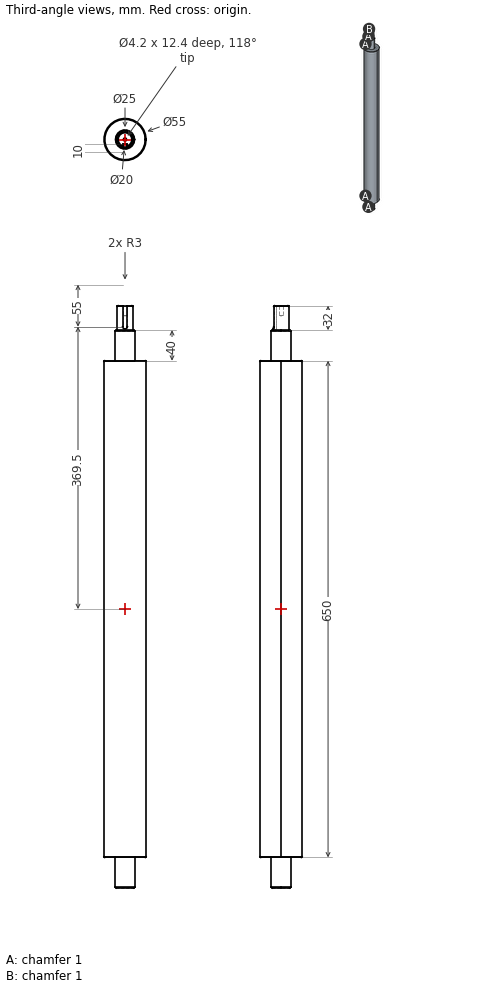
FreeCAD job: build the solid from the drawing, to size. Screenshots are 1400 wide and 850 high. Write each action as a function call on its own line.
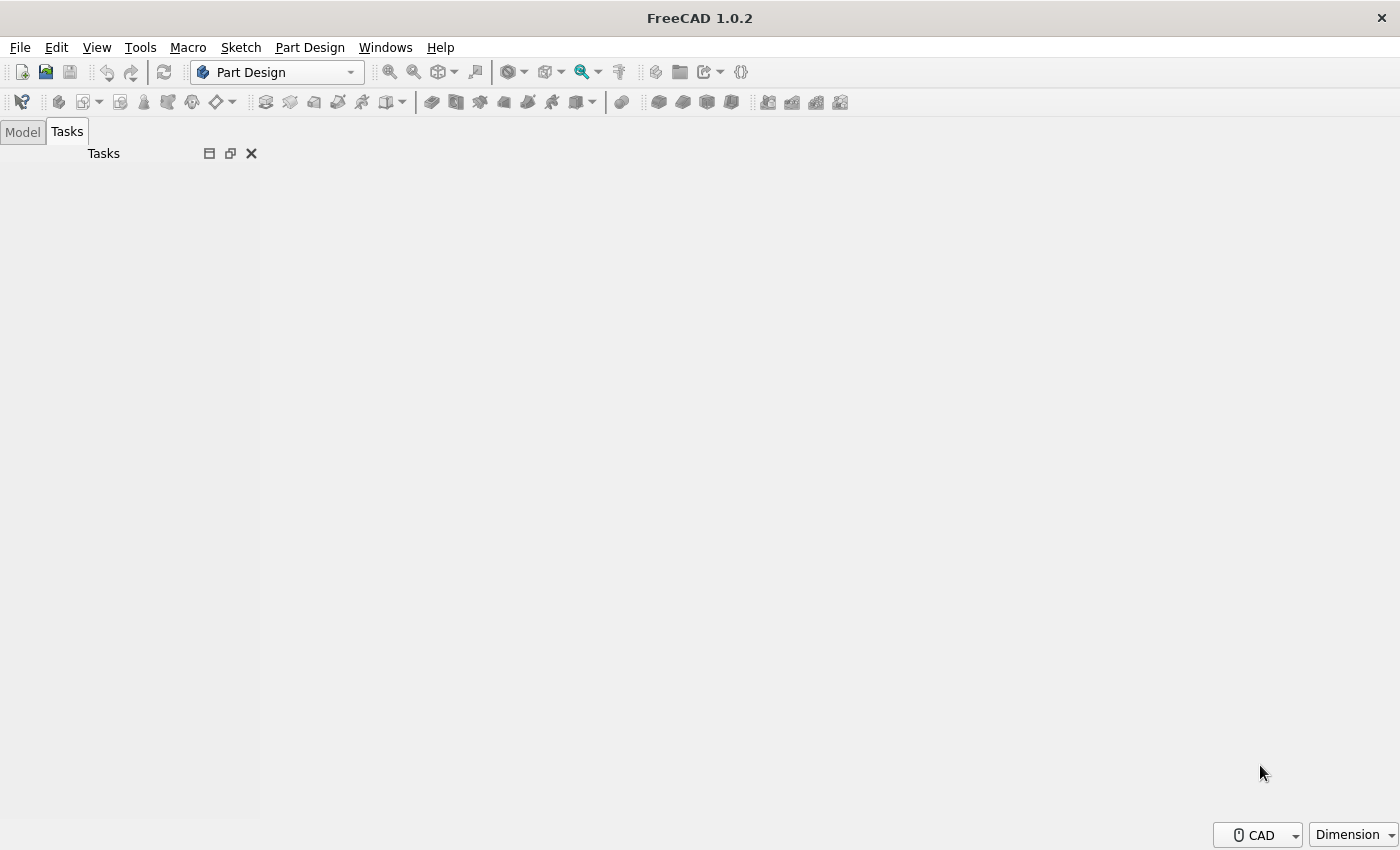
click(22, 72)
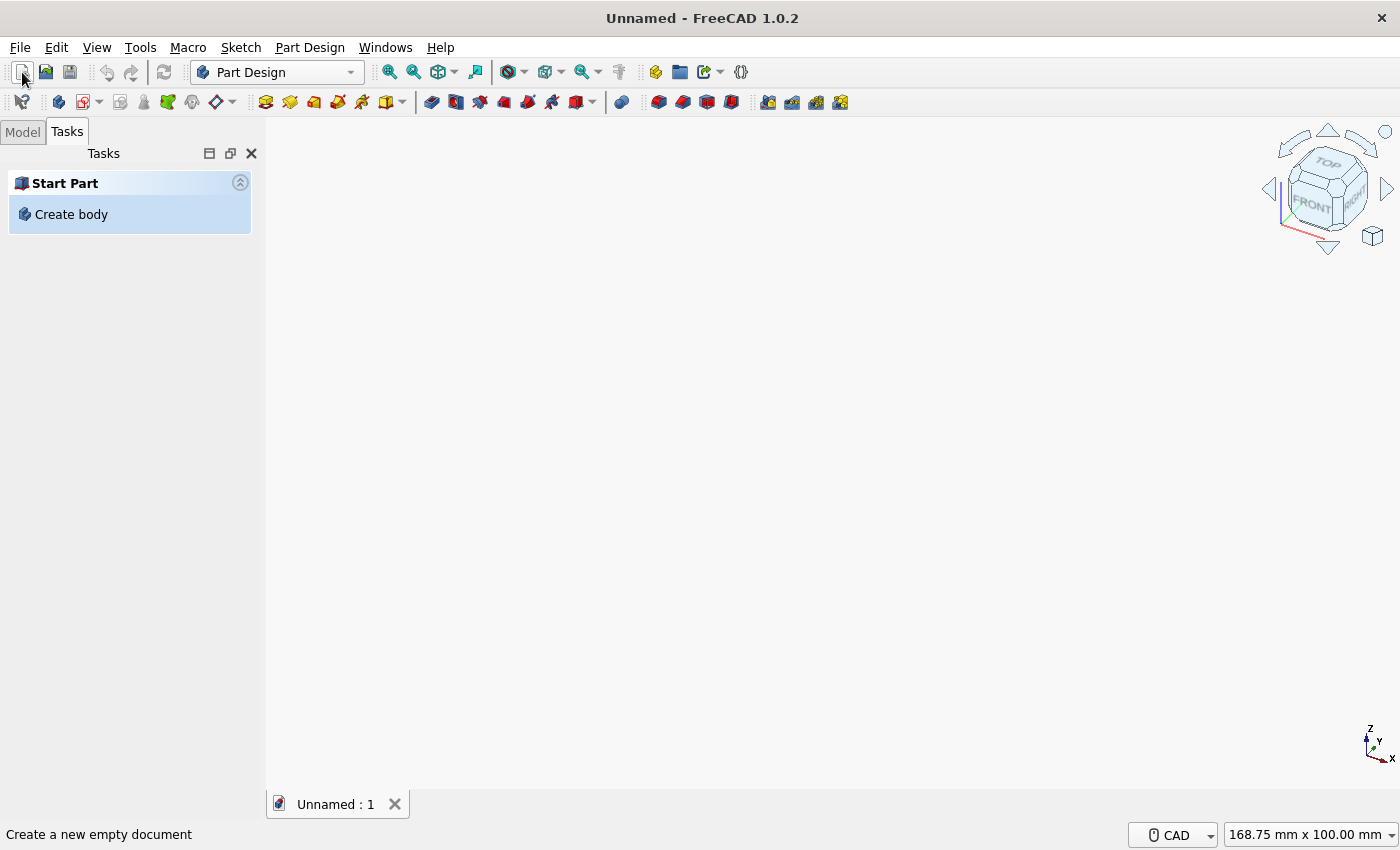
click(84, 102)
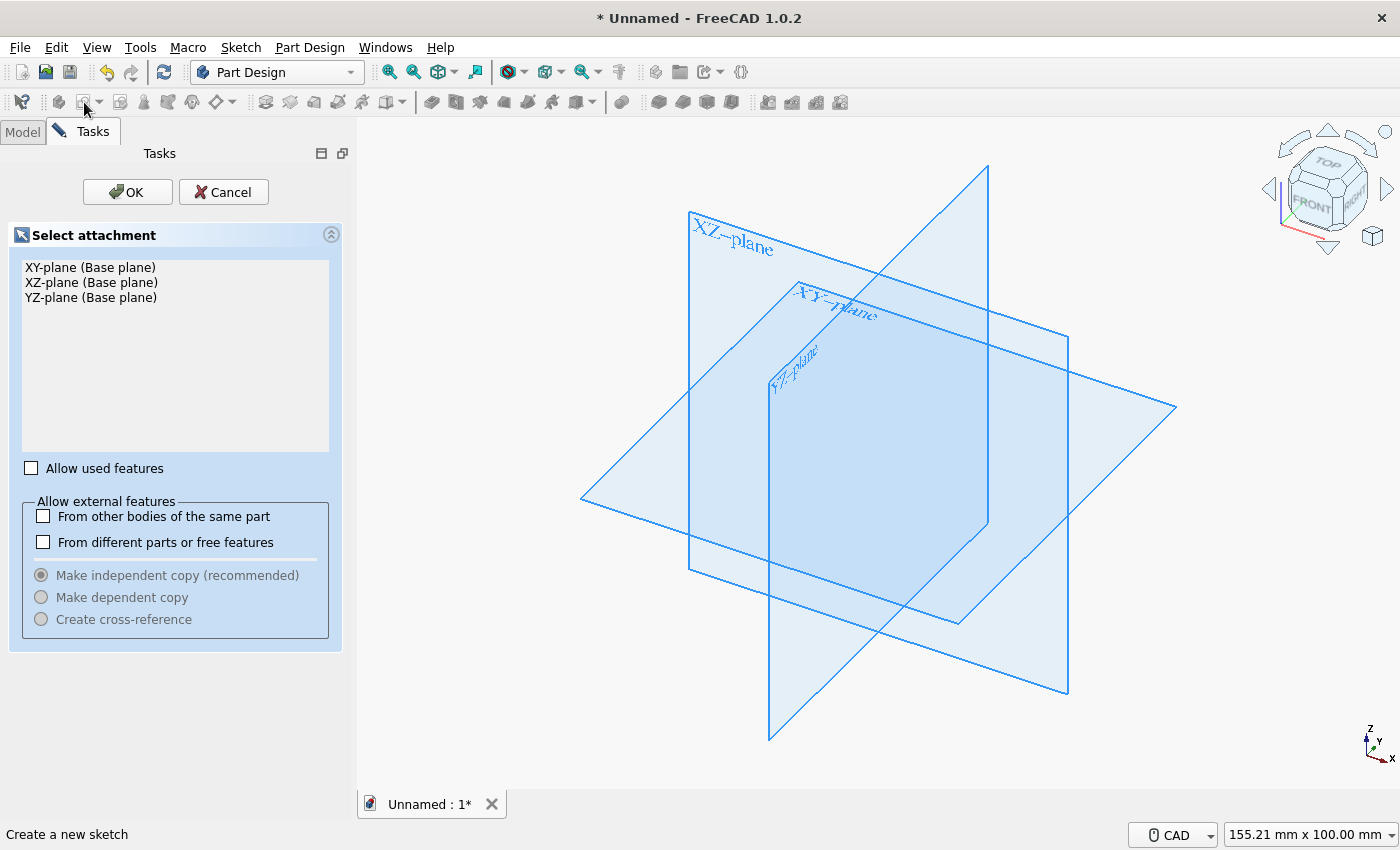
click(82, 268)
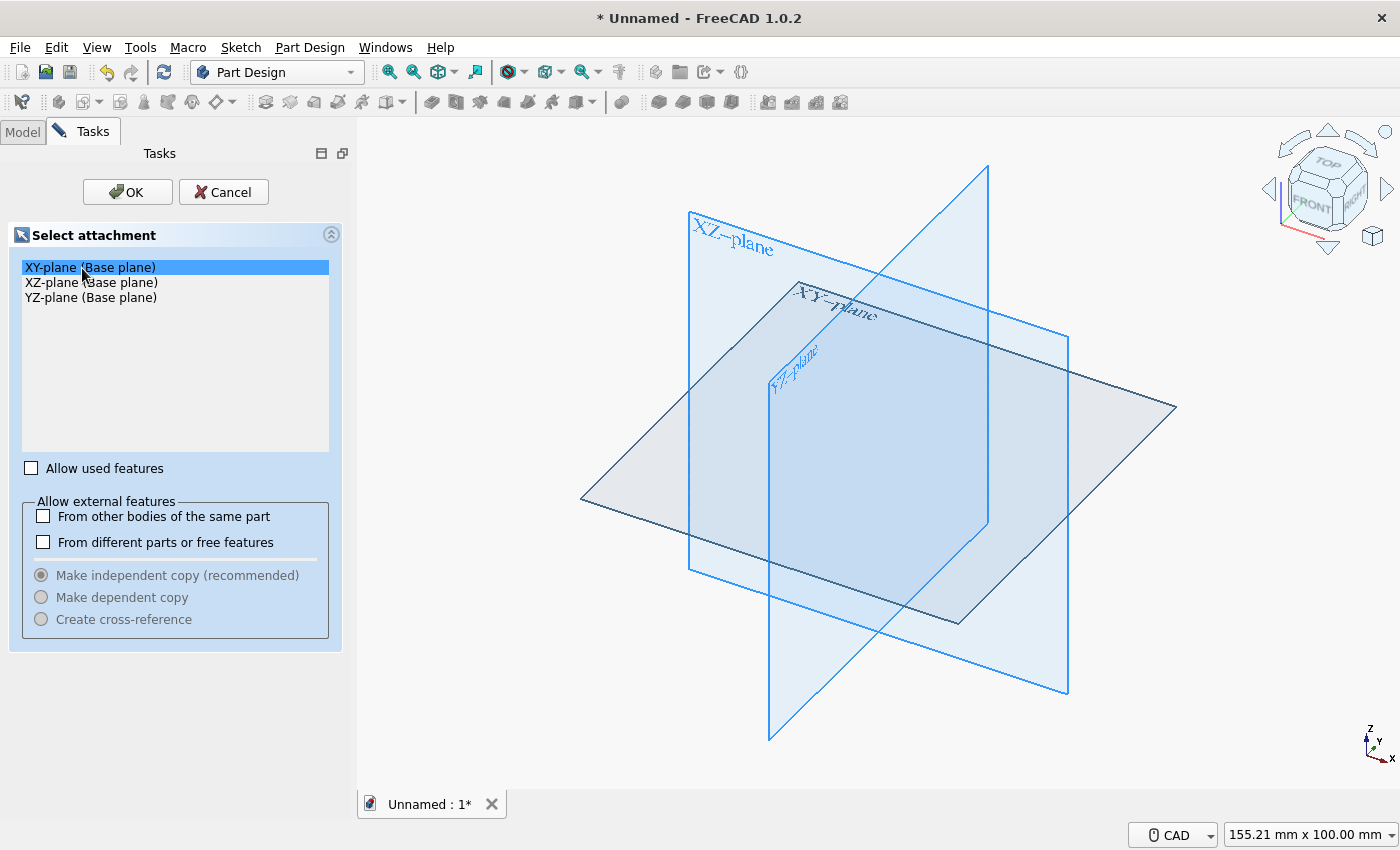
click(128, 192)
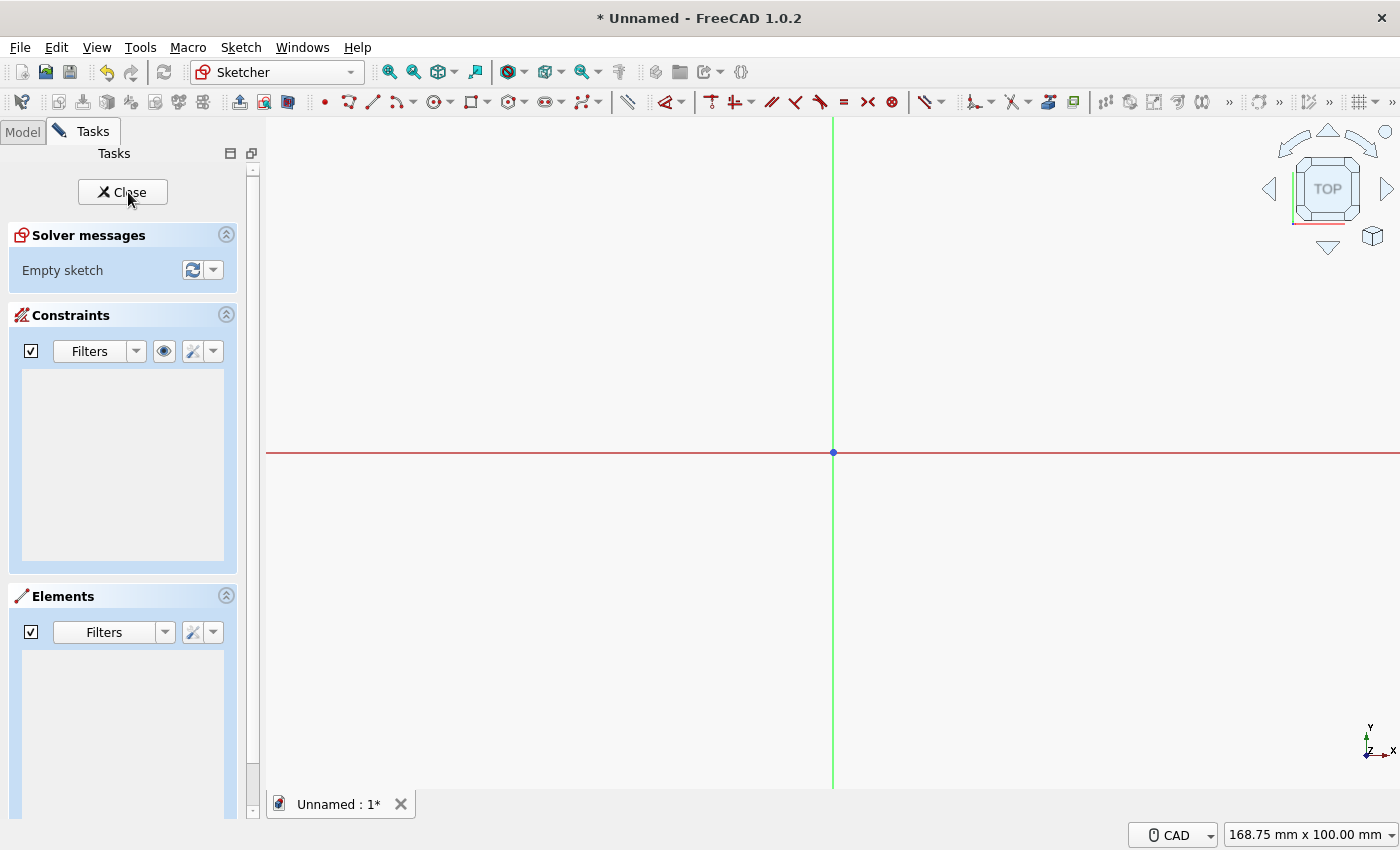
click(434, 102)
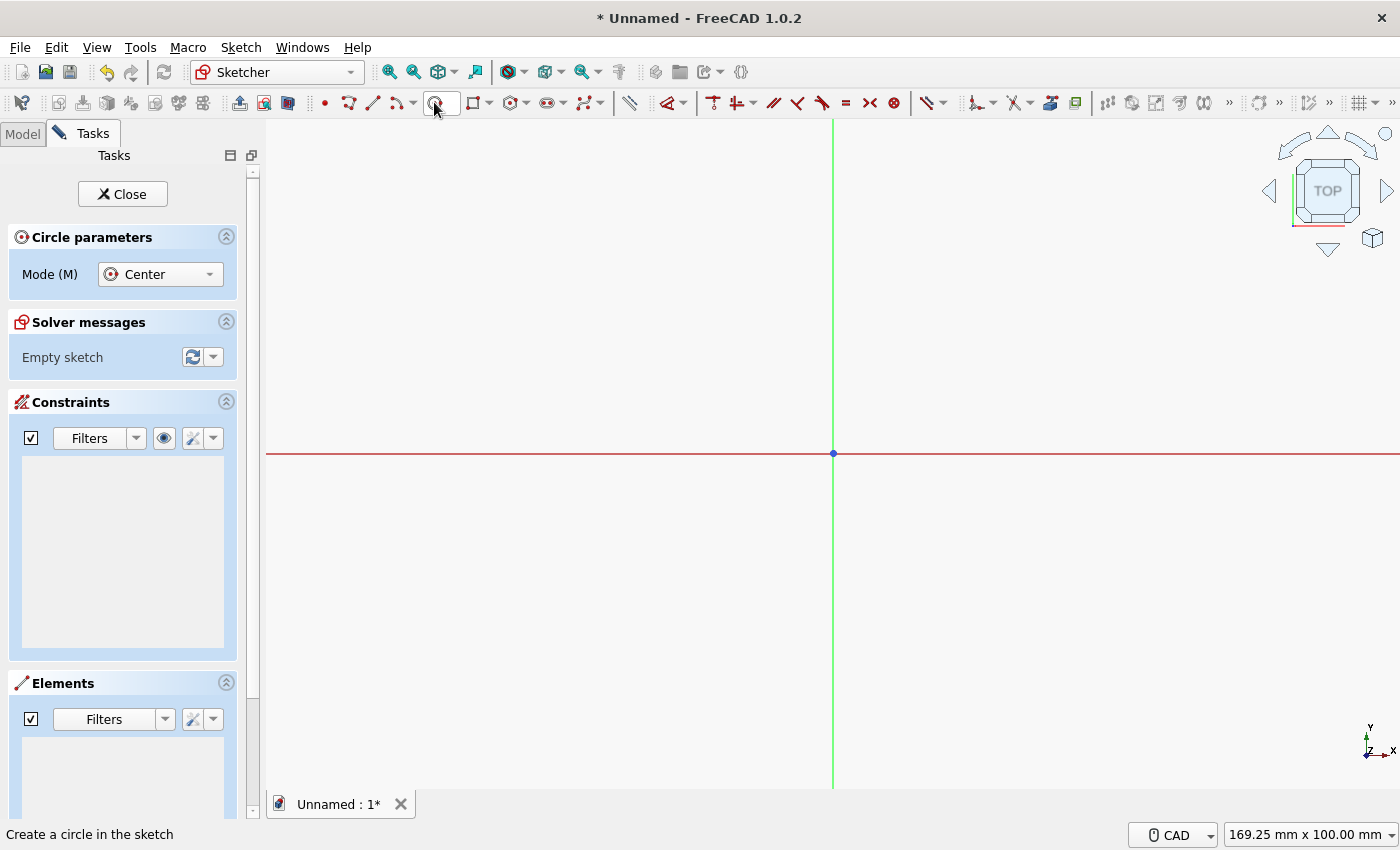
click(833, 454)
move(963, 324)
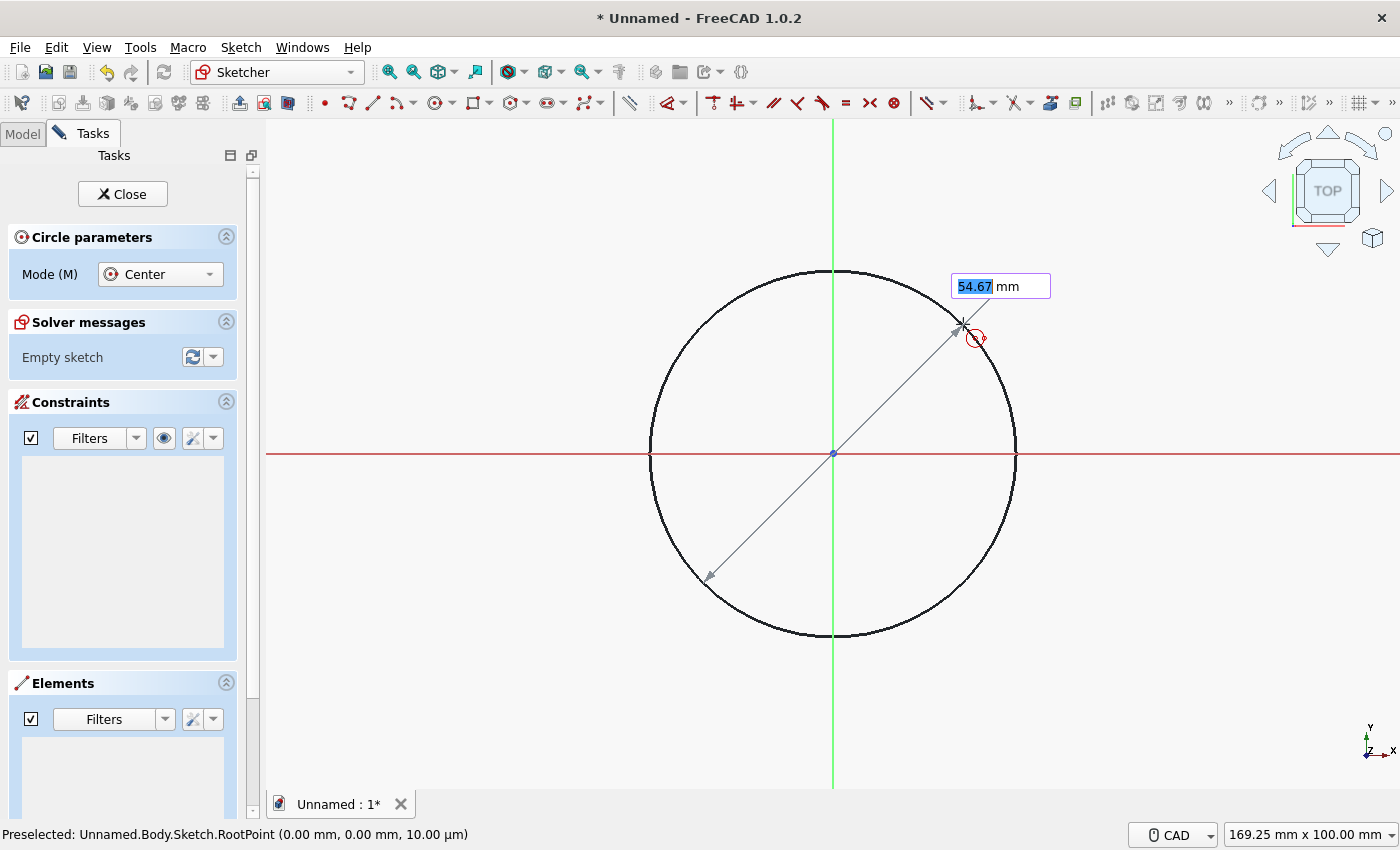
text(55)
key(Return)
key(Escape)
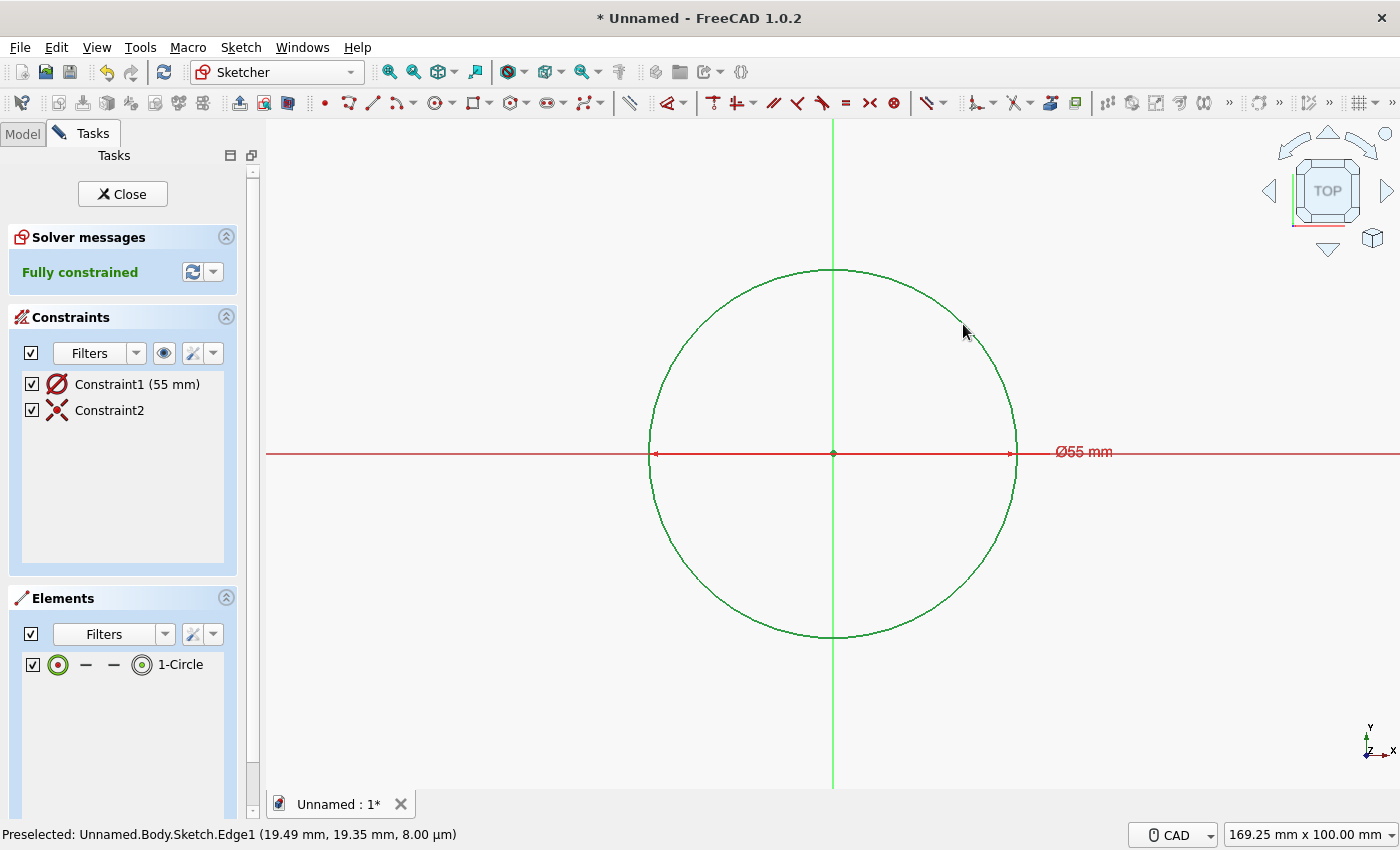
click(123, 194)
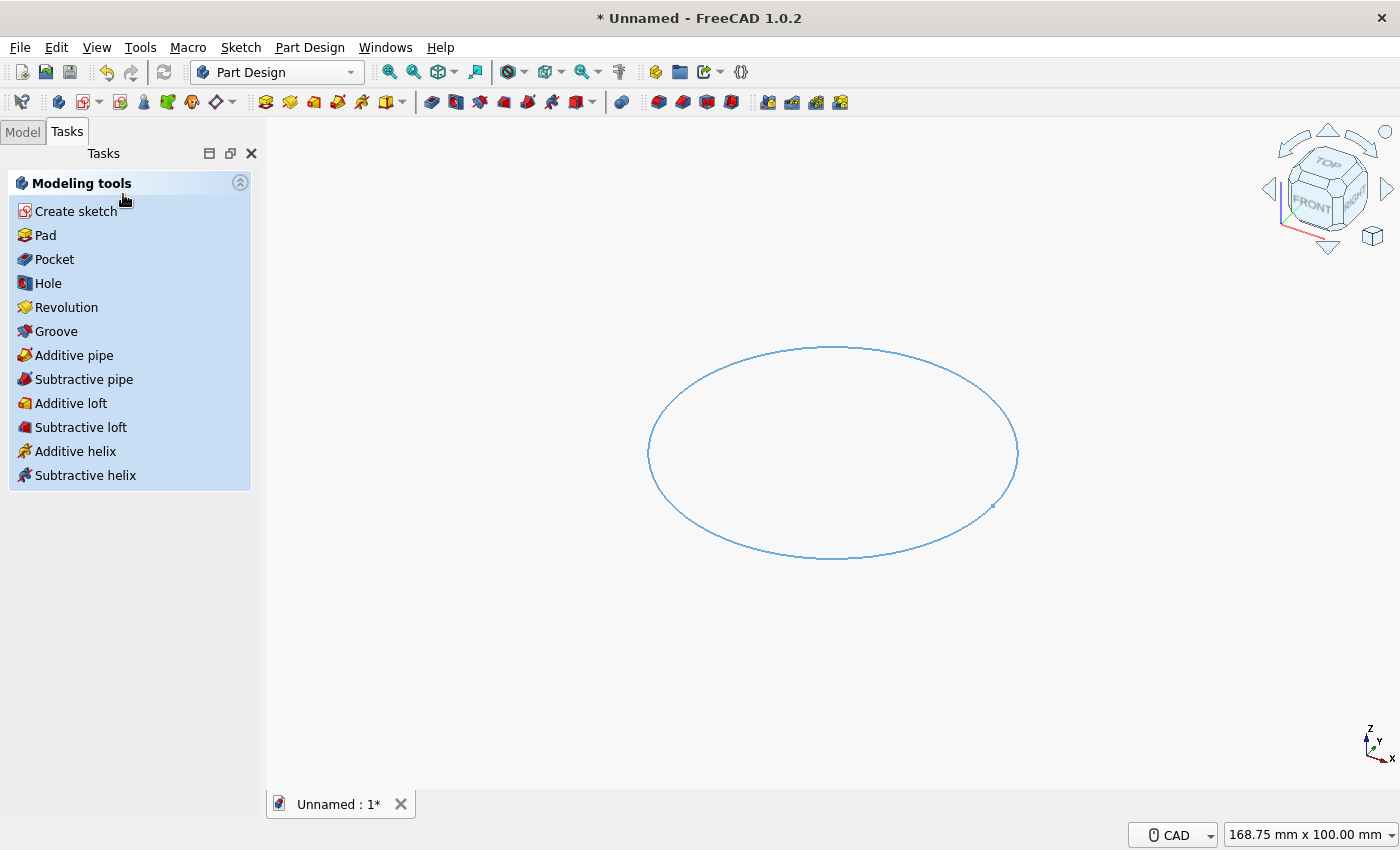
click(266, 102)